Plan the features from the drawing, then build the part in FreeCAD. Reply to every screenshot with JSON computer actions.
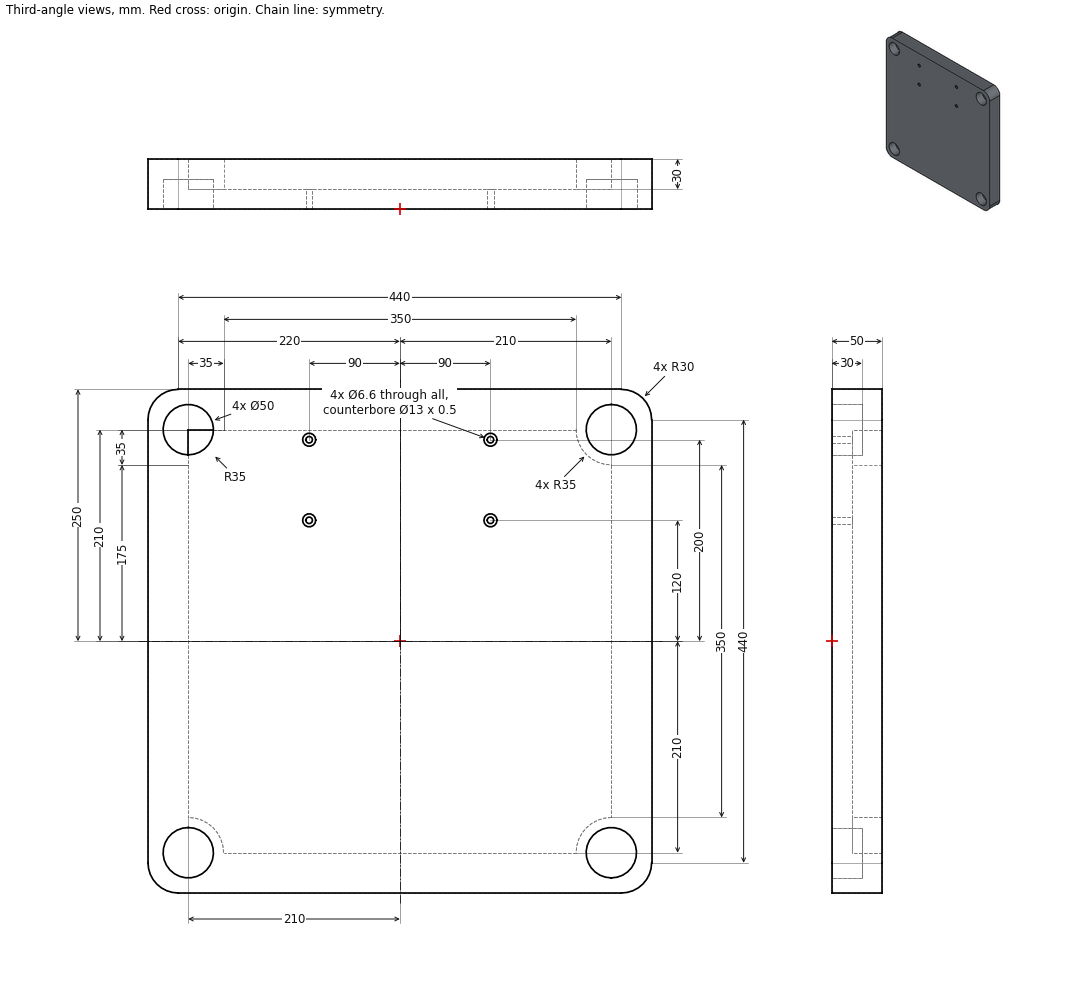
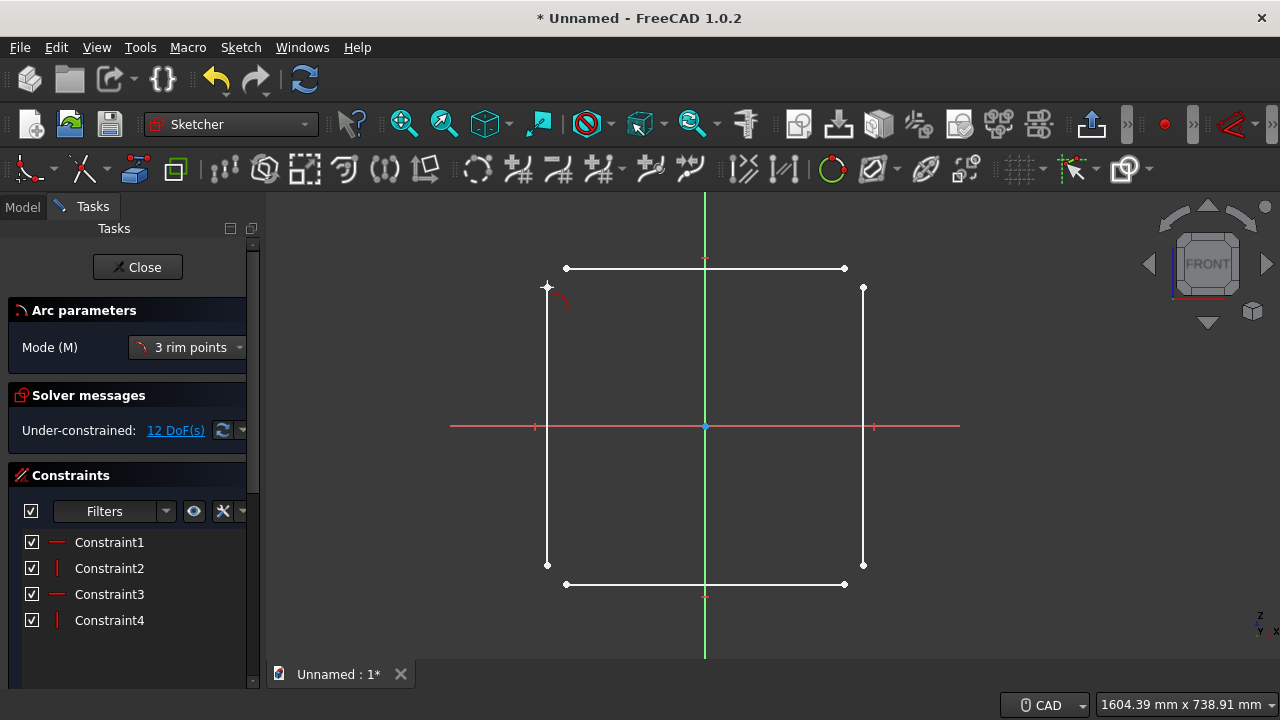
{"action": "left_click", "coordinate": [844, 269]}
{"action": "left_click", "coordinate": [863, 288]}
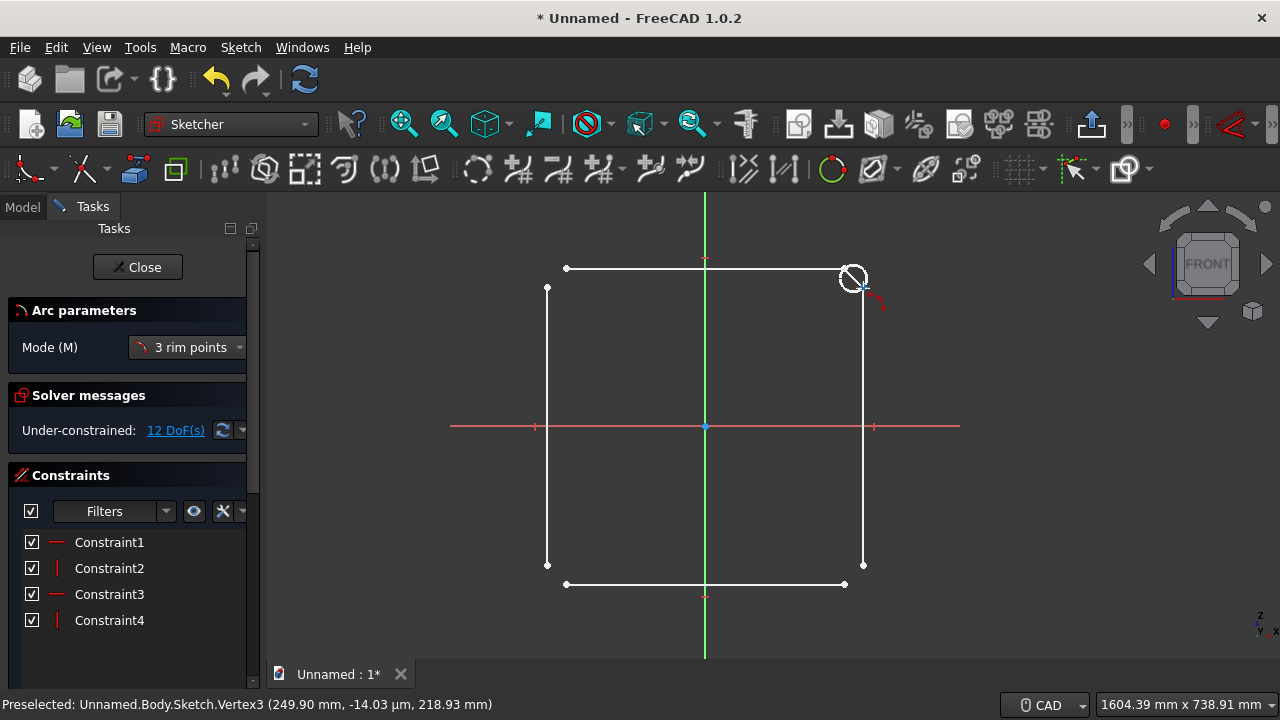
{"action": "scroll", "coordinate": [858, 274], "scroll_direction": "up", "scroll_amount": 6}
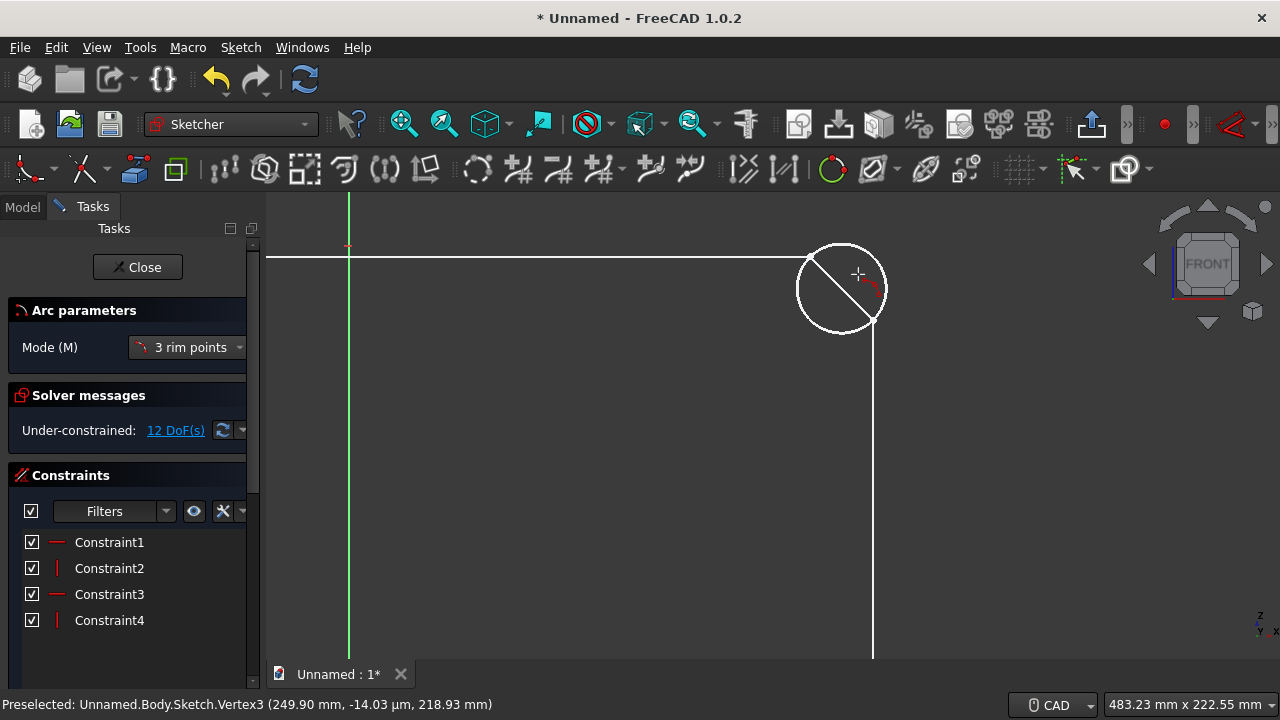
{"action": "left_click", "coordinate": [855, 273]}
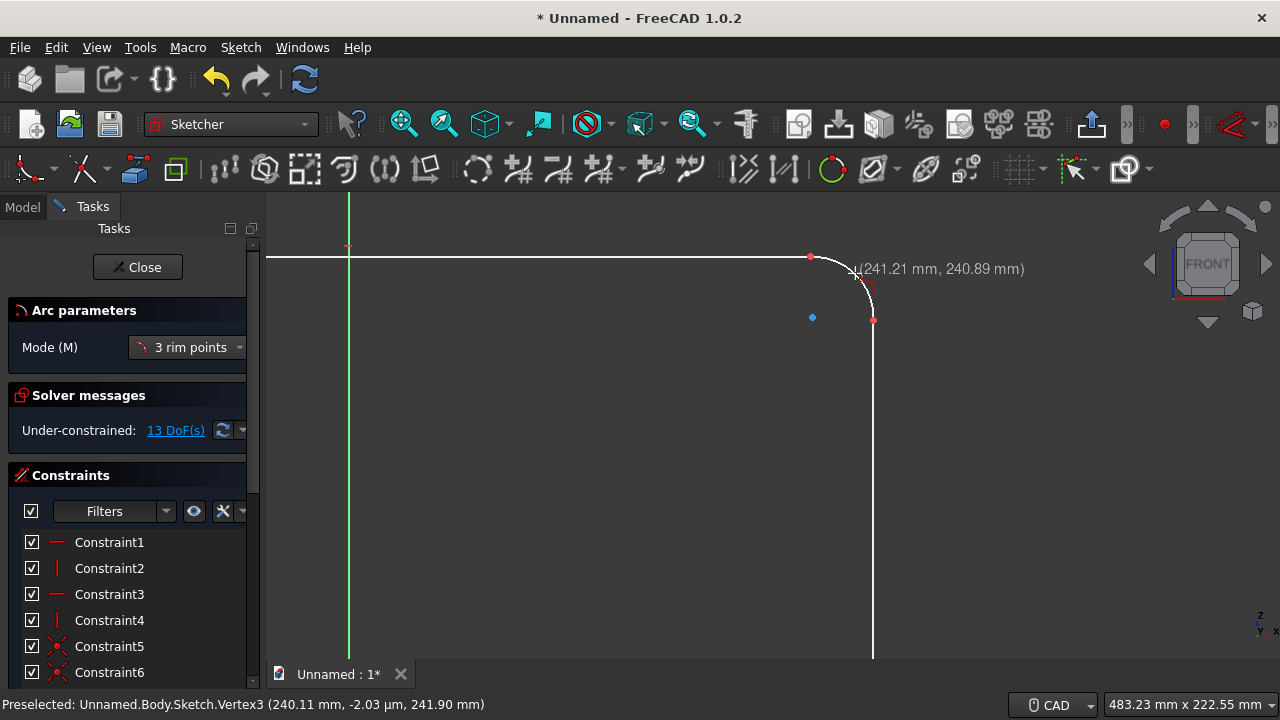
{"action": "scroll", "coordinate": [858, 273], "scroll_direction": "down", "scroll_amount": 6}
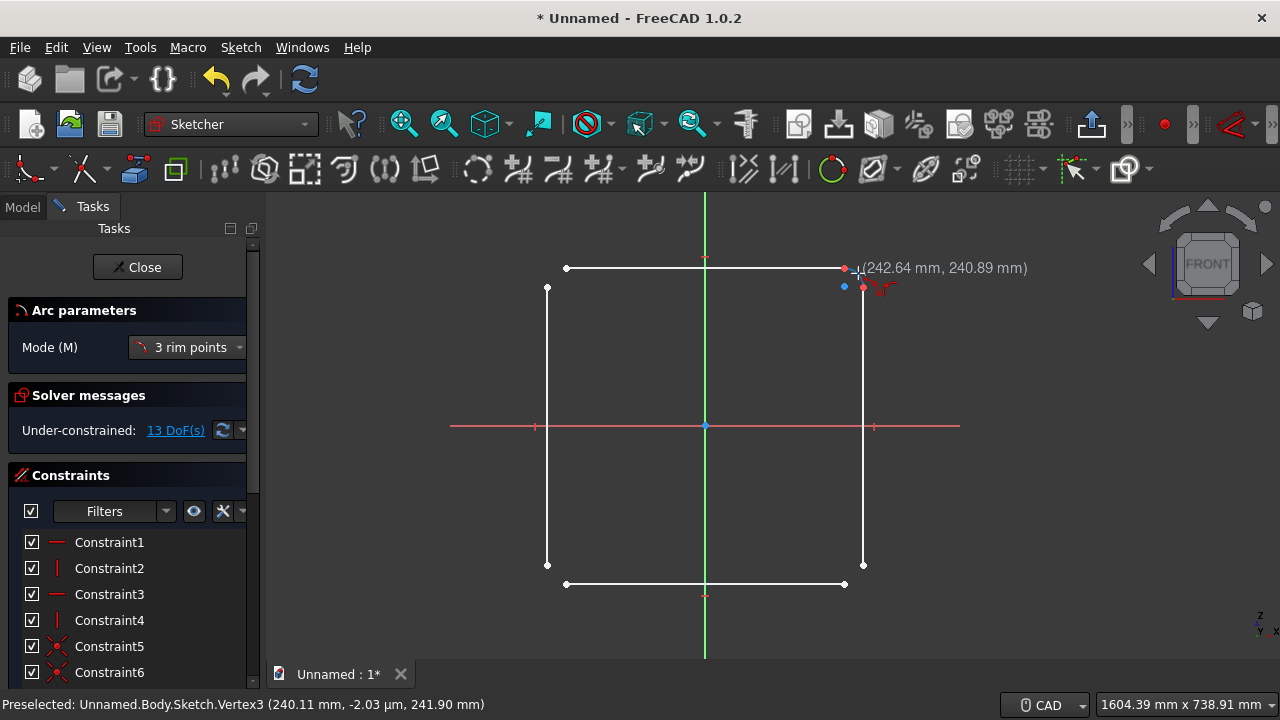
{"action": "left_click", "coordinate": [863, 565]}
{"action": "left_click", "coordinate": [844, 584]}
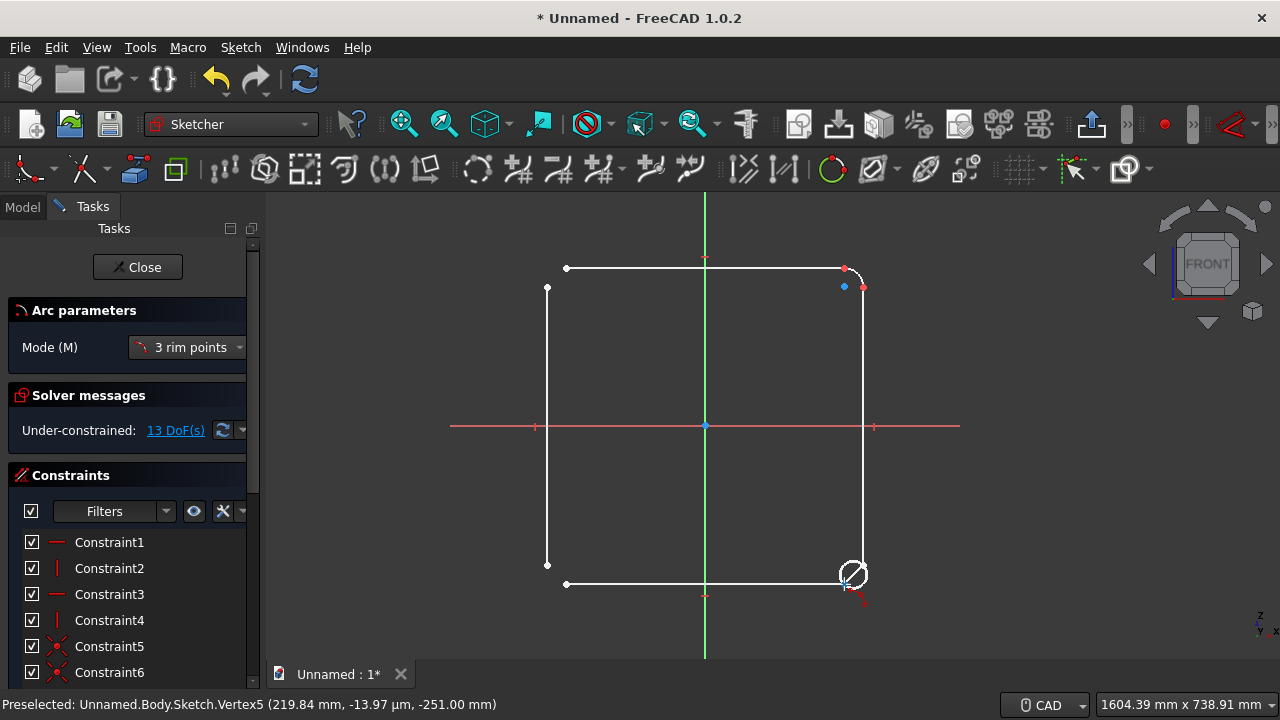
{"action": "scroll", "coordinate": [858, 578], "scroll_direction": "up", "scroll_amount": 6}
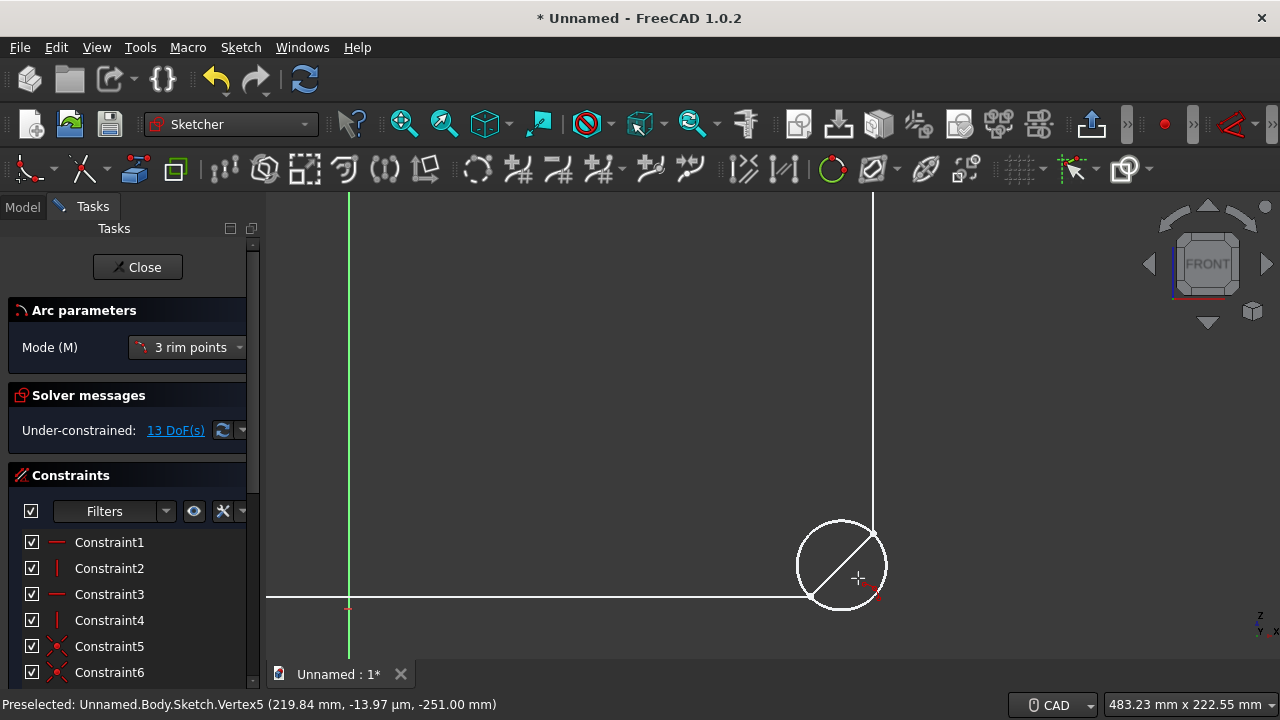
{"action": "left_click", "coordinate": [855, 576]}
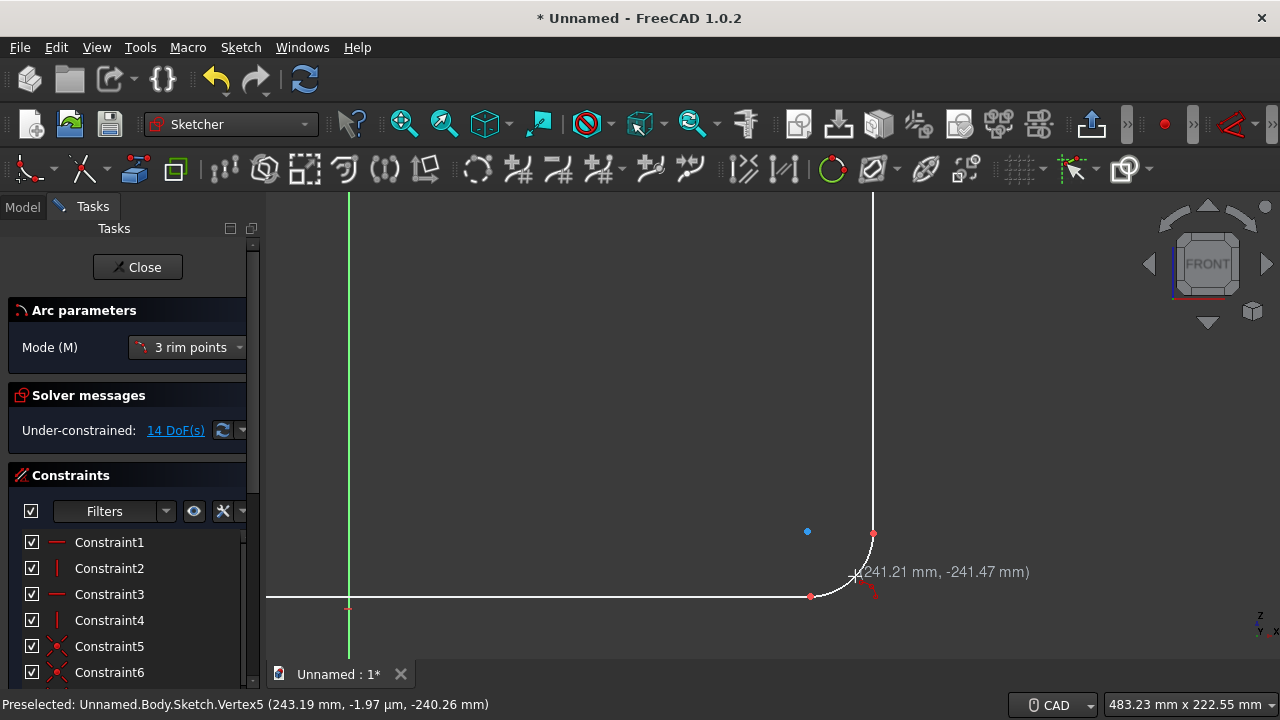
{"action": "scroll", "coordinate": [858, 579], "scroll_direction": "down", "scroll_amount": 6}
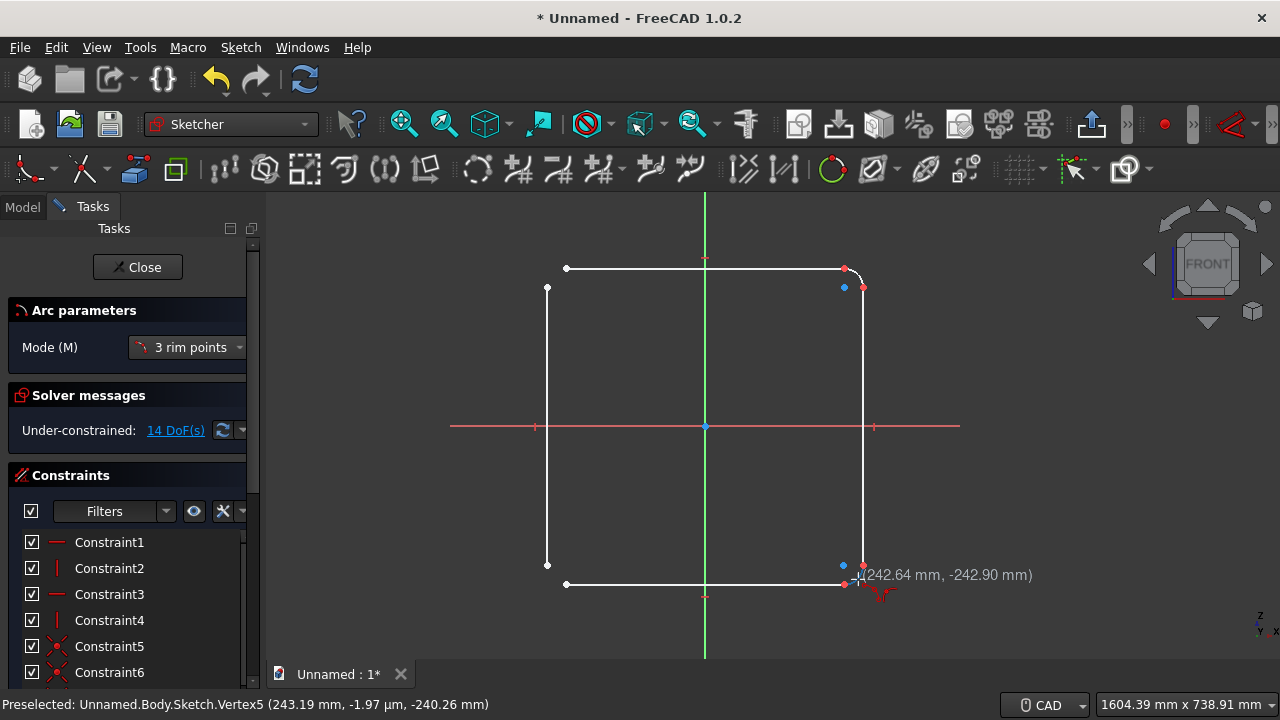
{"action": "left_click", "coordinate": [566, 585]}
{"action": "left_click", "coordinate": [547, 566]}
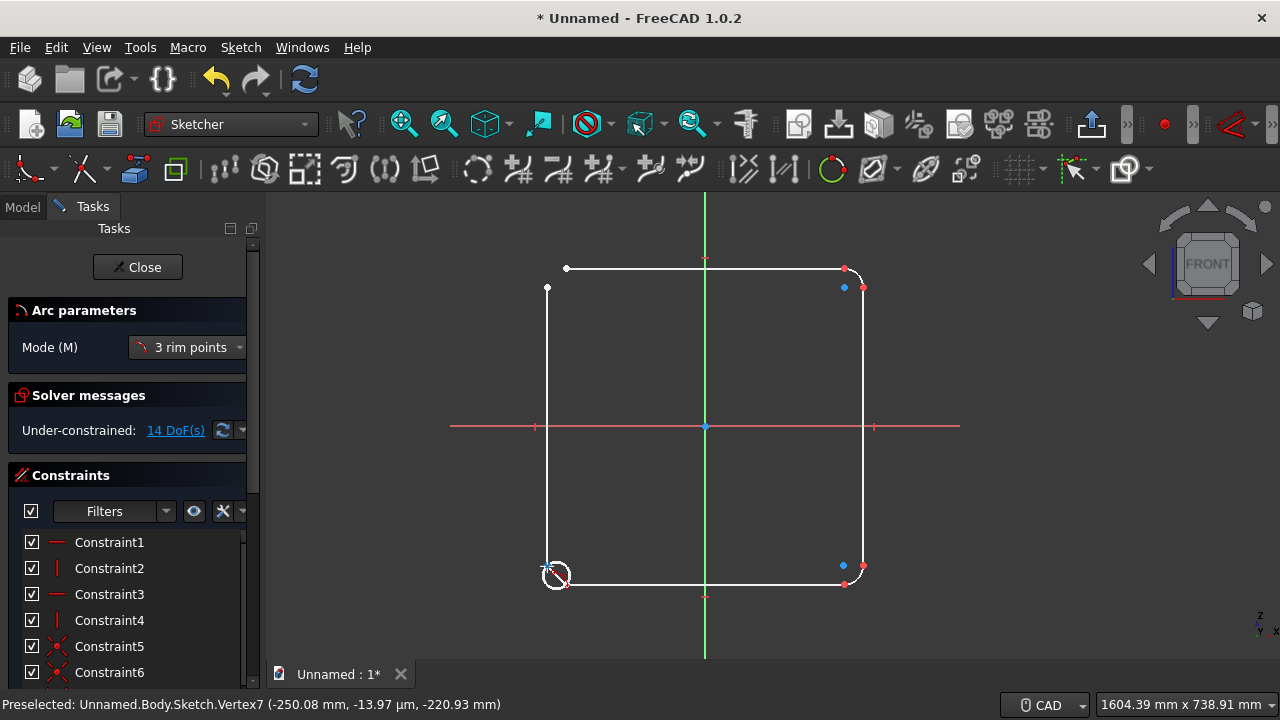
{"action": "scroll", "coordinate": [553, 579], "scroll_direction": "up", "scroll_amount": 6}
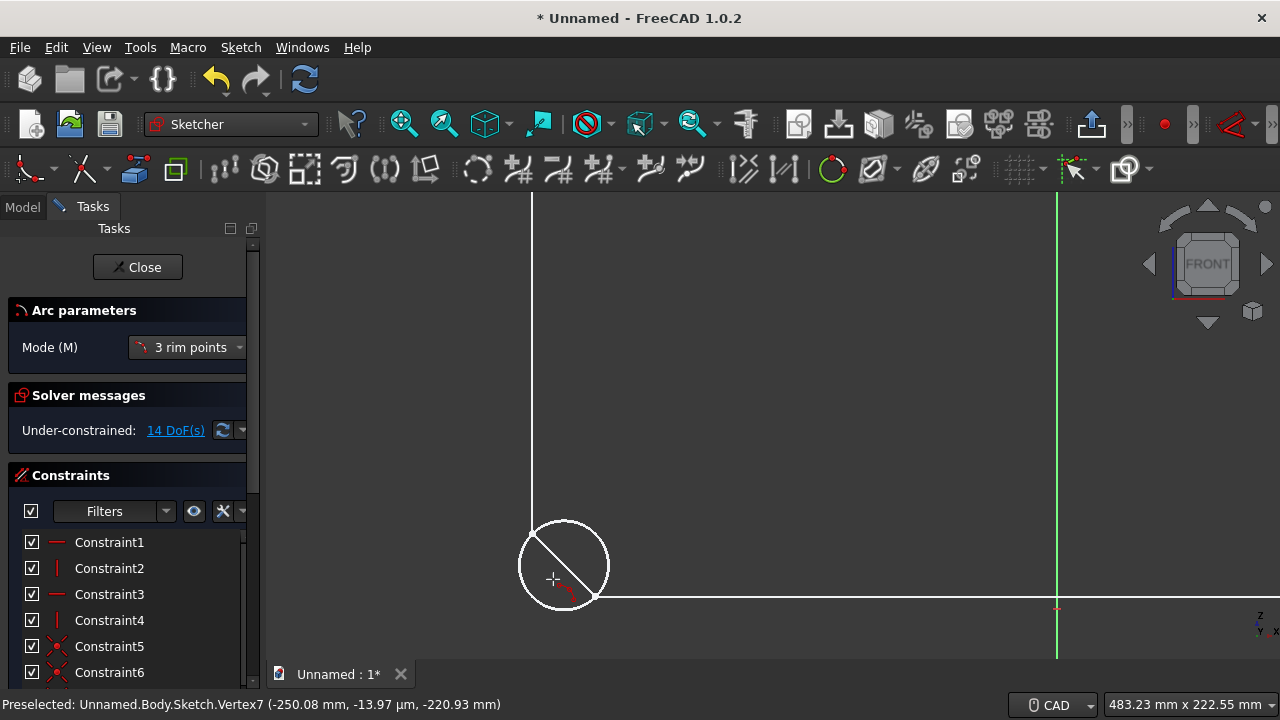
{"action": "left_click", "coordinate": [551, 576]}